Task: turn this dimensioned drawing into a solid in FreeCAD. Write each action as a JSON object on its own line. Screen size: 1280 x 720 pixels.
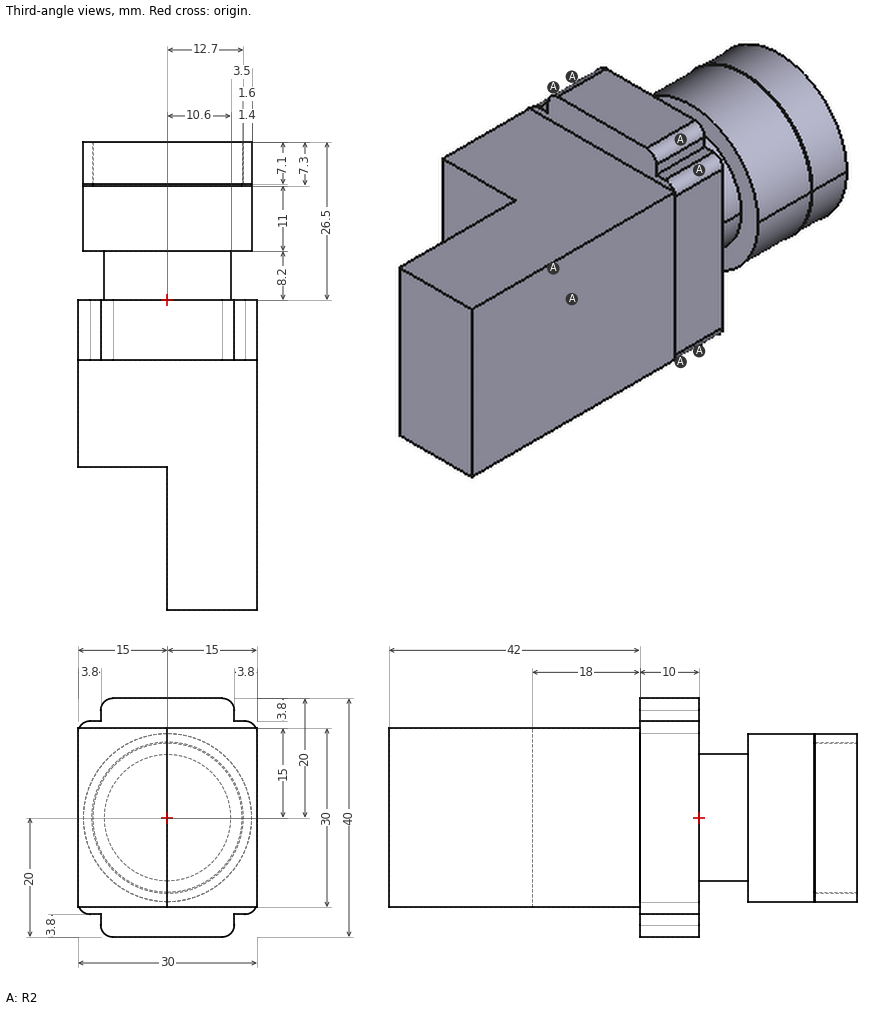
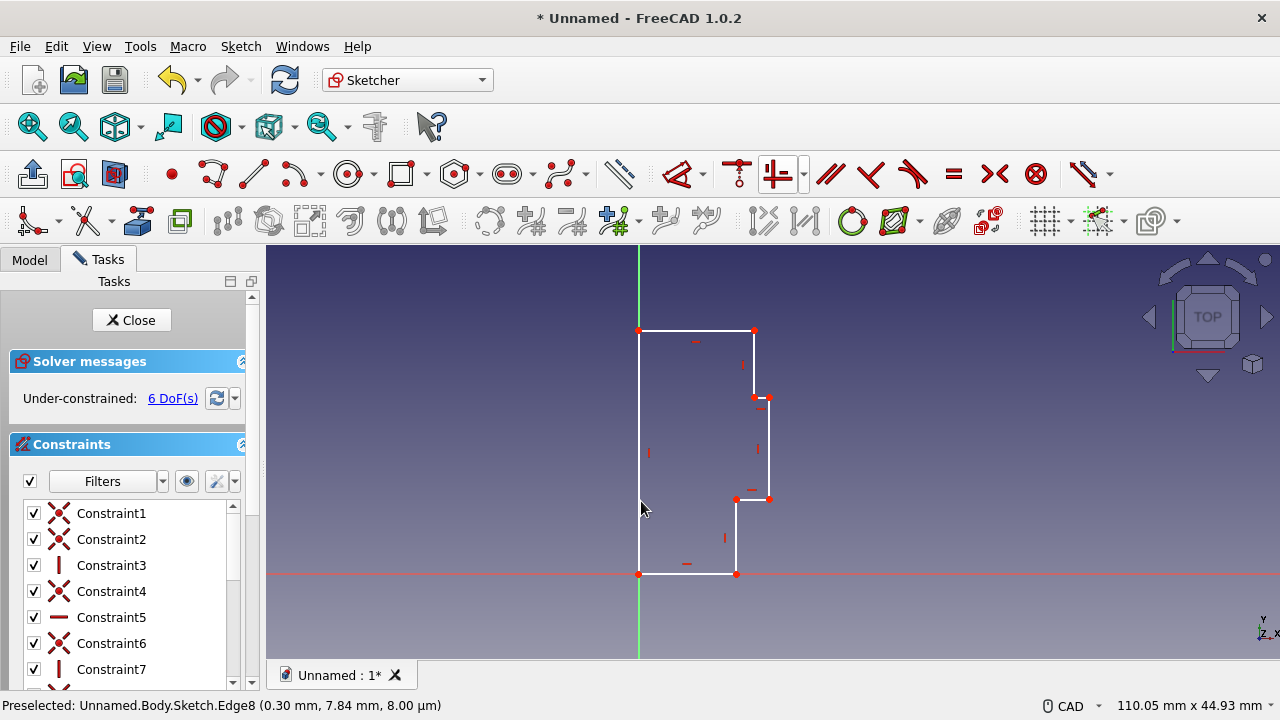
{"action": "key", "text": "d"}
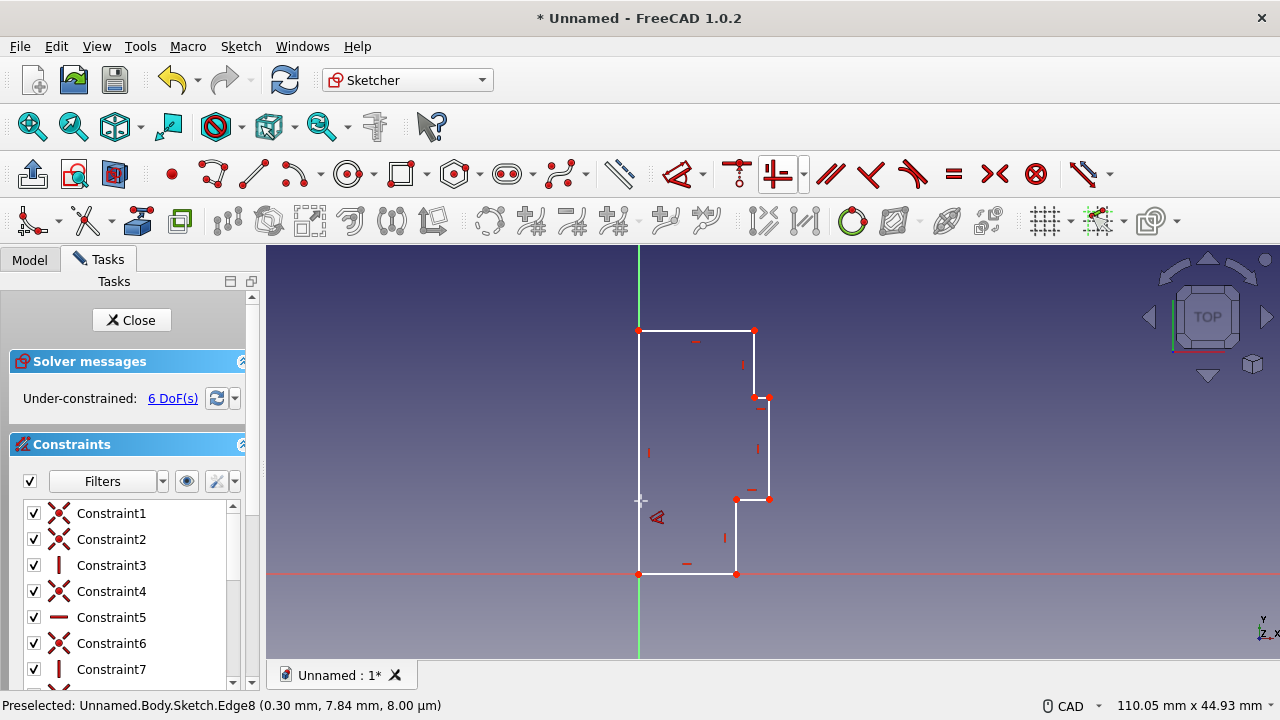
{"action": "left_click", "coordinate": [769, 469]}
{"action": "left_click", "coordinate": [803, 449]}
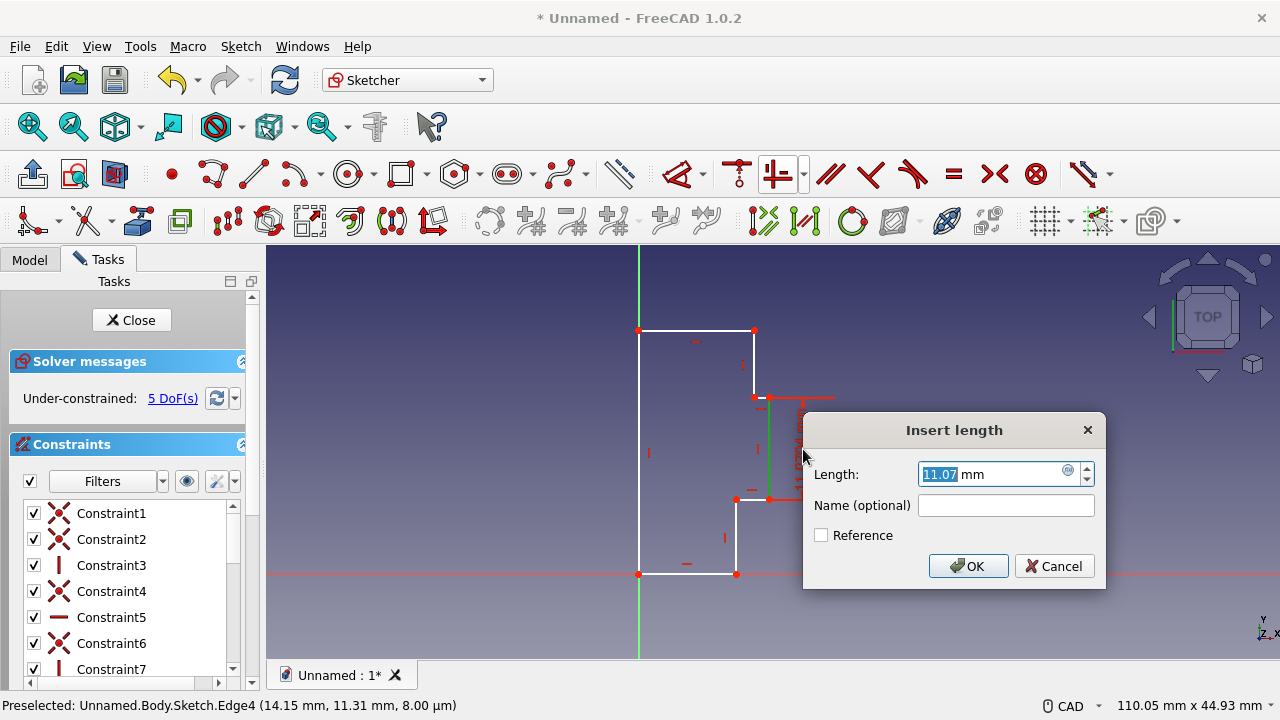
{"action": "type", "text": "11"}
{"action": "key", "text": "Return"}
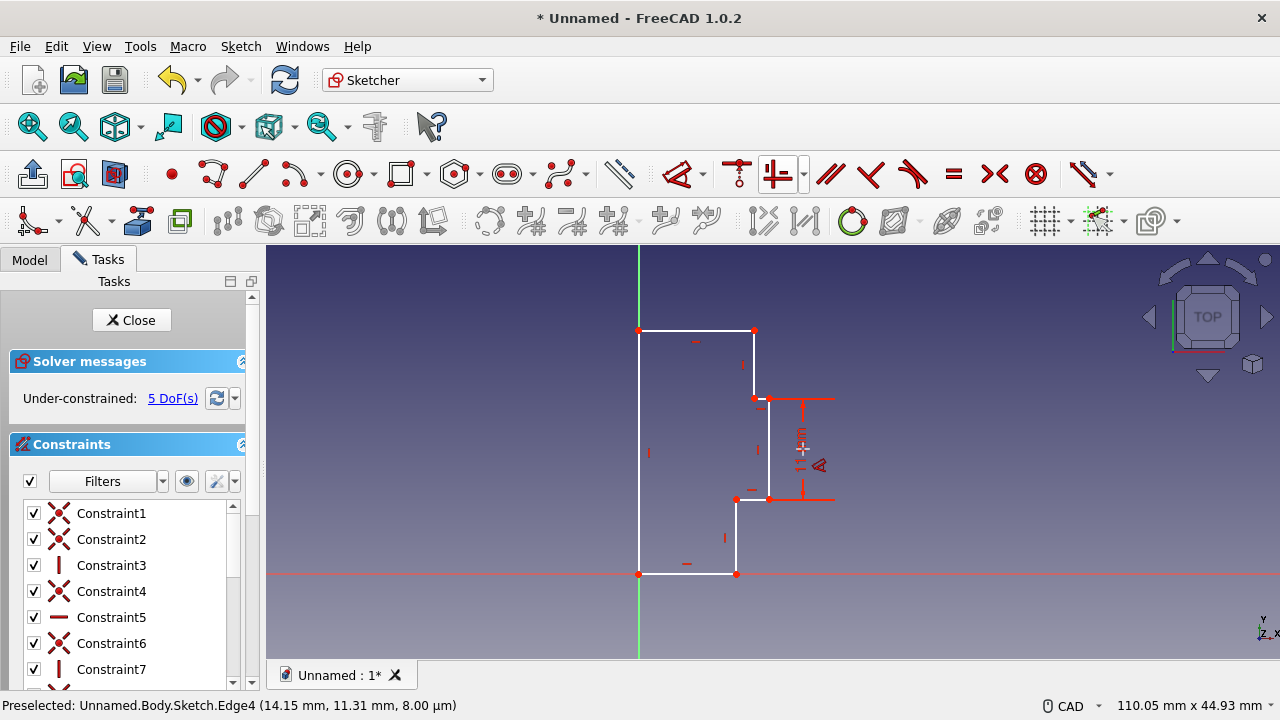
{"action": "left_click", "coordinate": [736, 552]}
{"action": "left_click", "coordinate": [770, 537]}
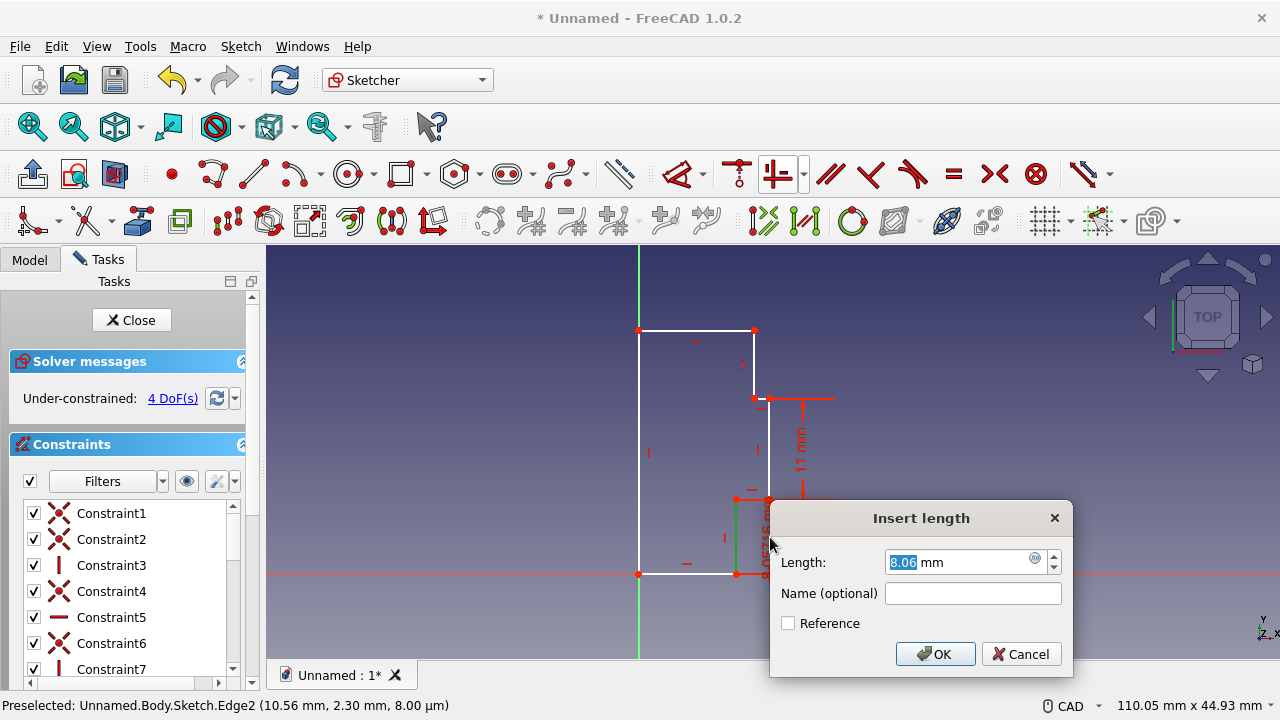
{"action": "type", "text": "8.2"}
{"action": "key", "text": "Return"}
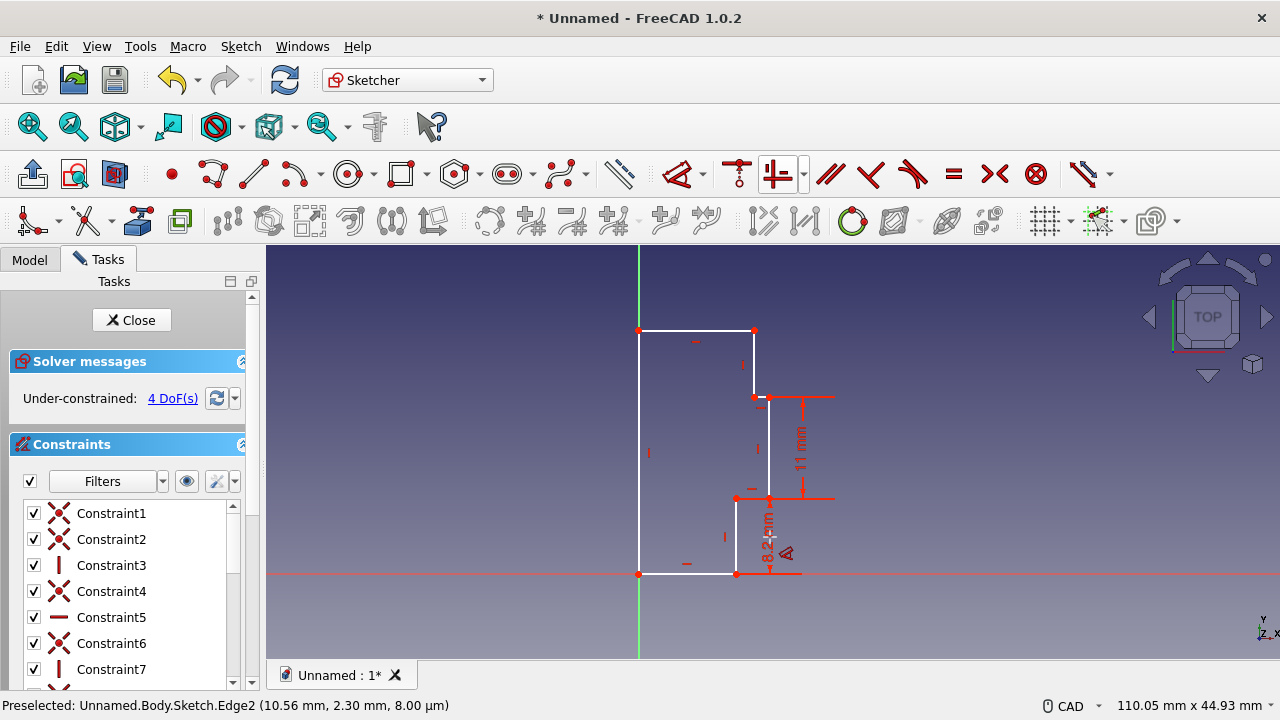
{"action": "scroll", "coordinate": [746, 499], "scroll_direction": "up", "scroll_amount": 2}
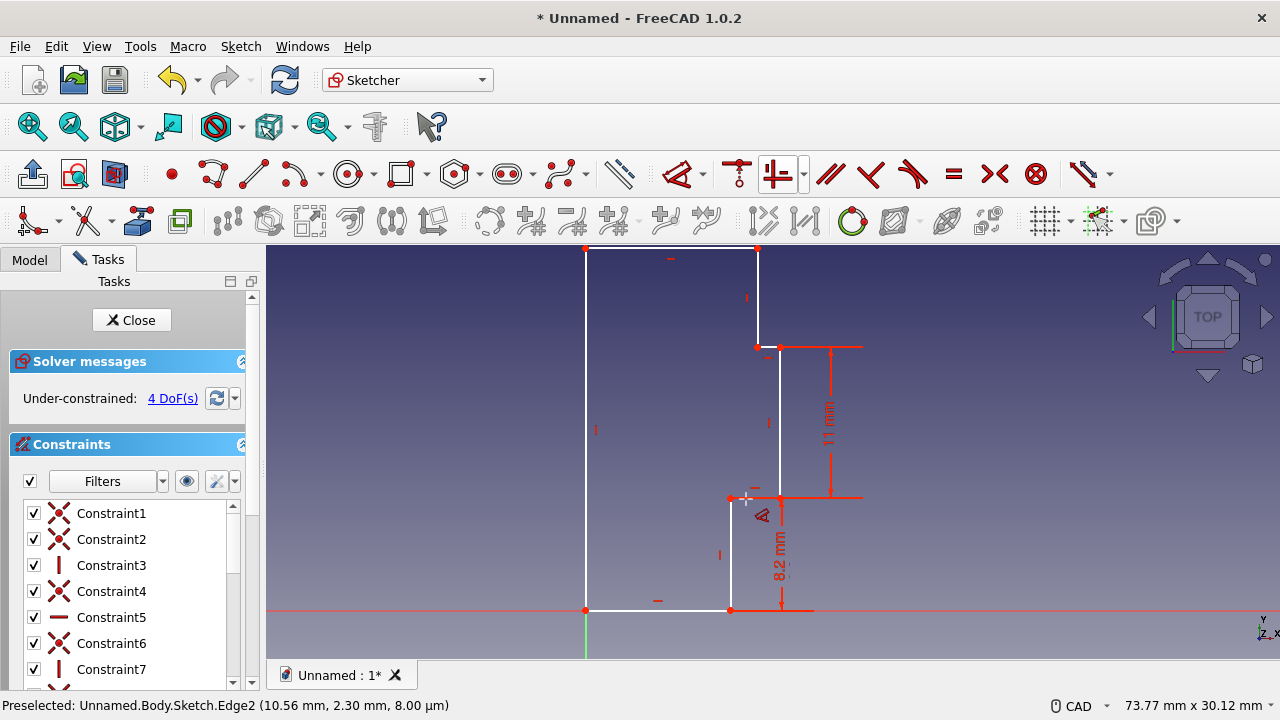
{"action": "left_click", "coordinate": [746, 498]}
{"action": "left_click", "coordinate": [755, 532]}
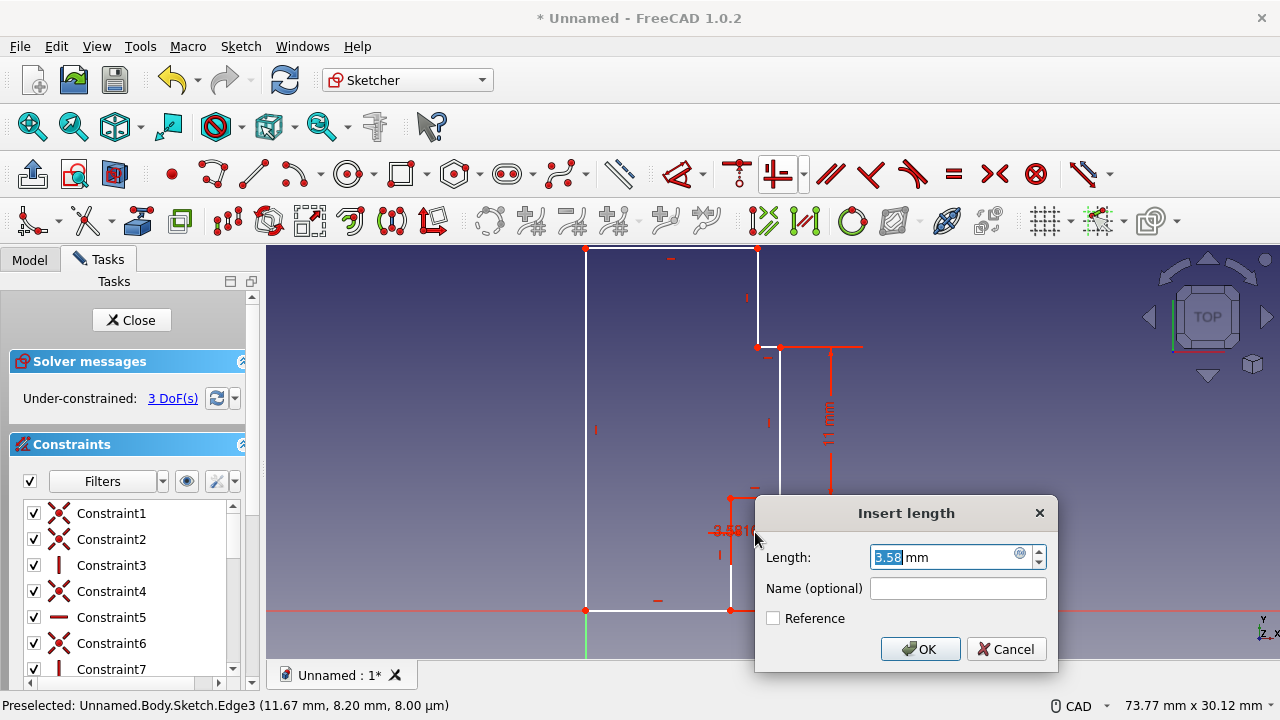
{"action": "type", "text": "3.5"}
{"action": "key", "text": "Return"}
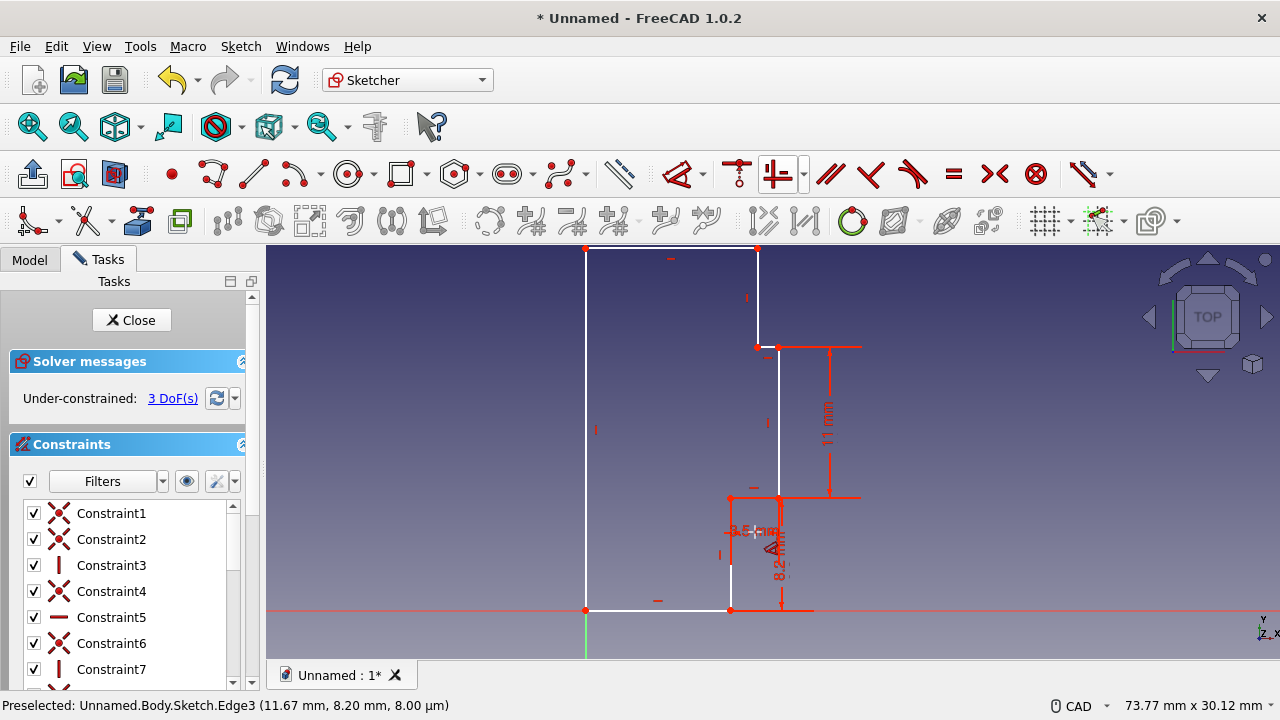
{"action": "scroll", "coordinate": [768, 347], "scroll_direction": "up", "scroll_amount": 3}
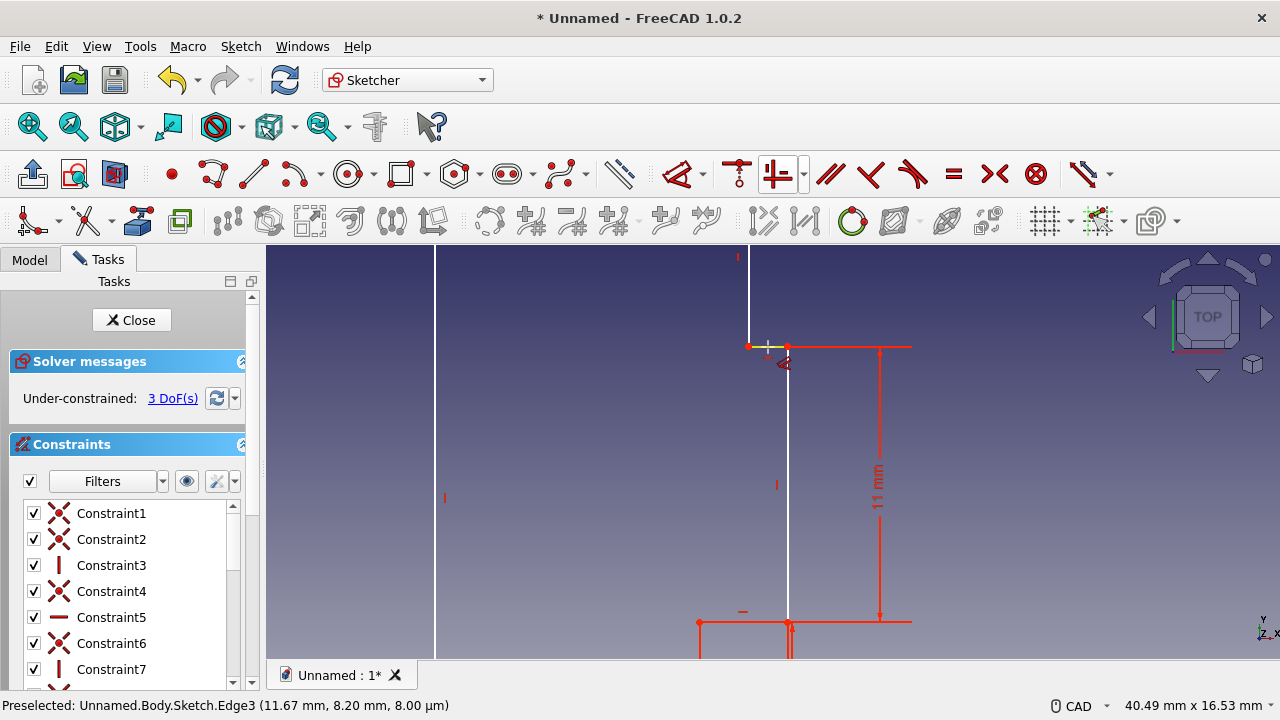
{"action": "left_click", "coordinate": [768, 347]}
{"action": "left_click", "coordinate": [768, 313]}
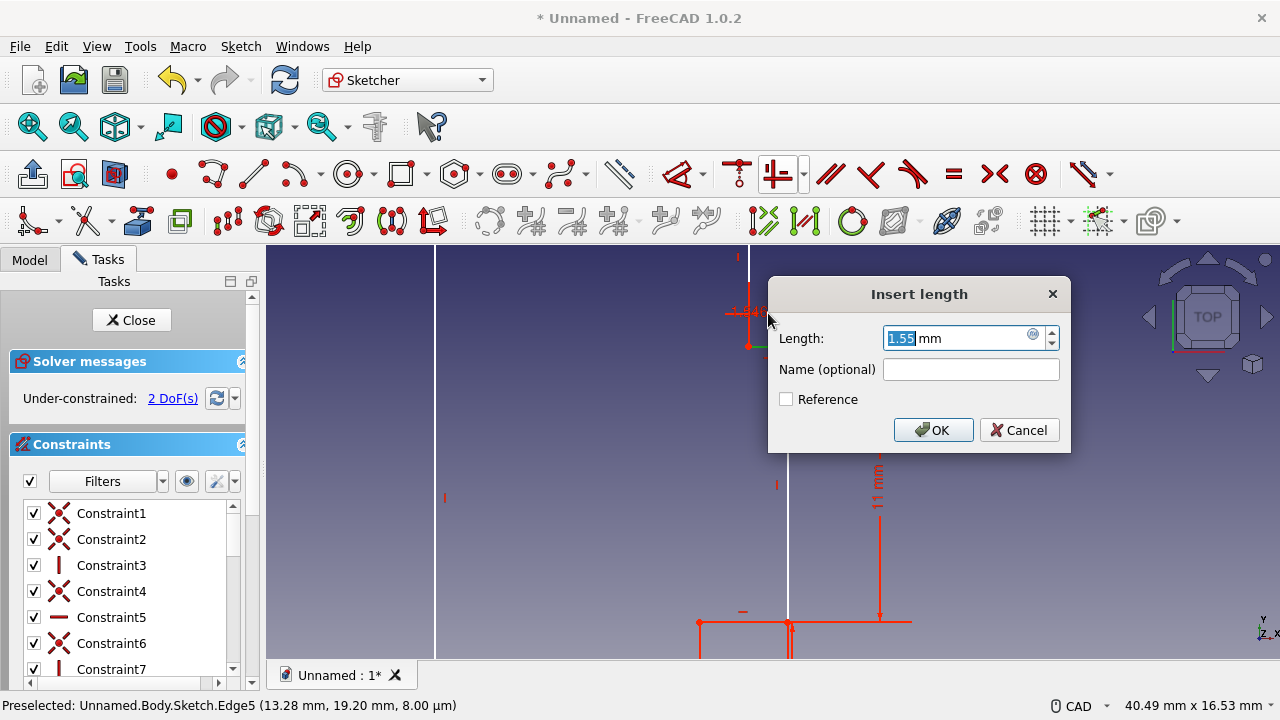
{"action": "type", "text": "1.6"}
{"action": "key", "text": "Return"}